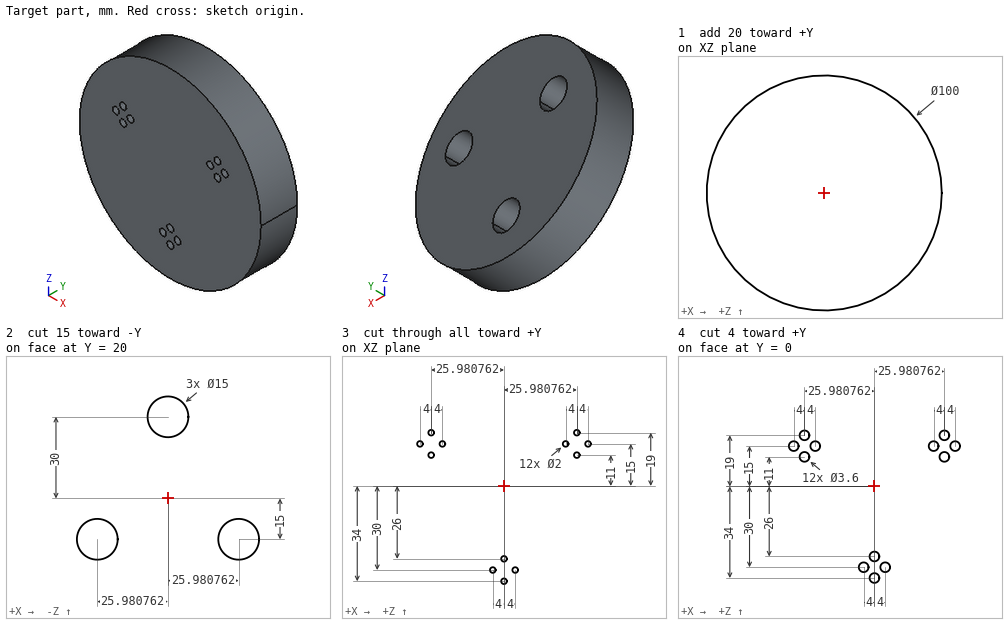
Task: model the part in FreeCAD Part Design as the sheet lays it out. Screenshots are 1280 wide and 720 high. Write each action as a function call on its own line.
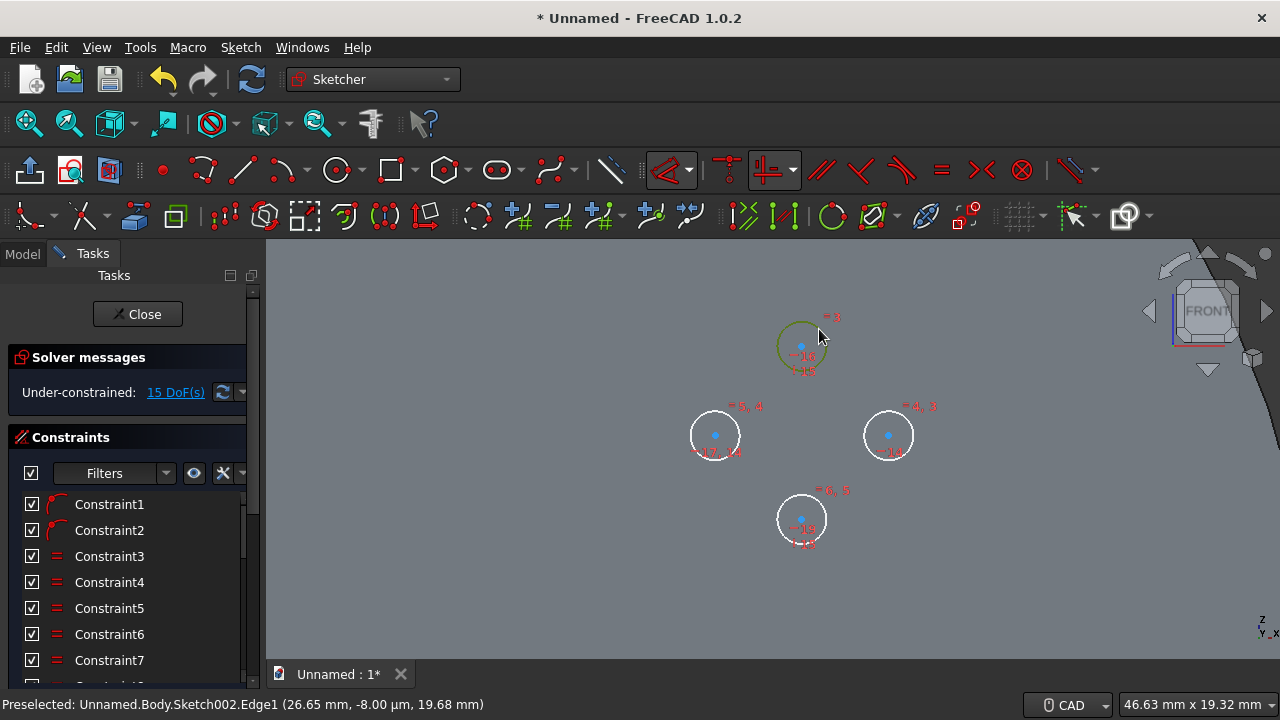
click(692, 170)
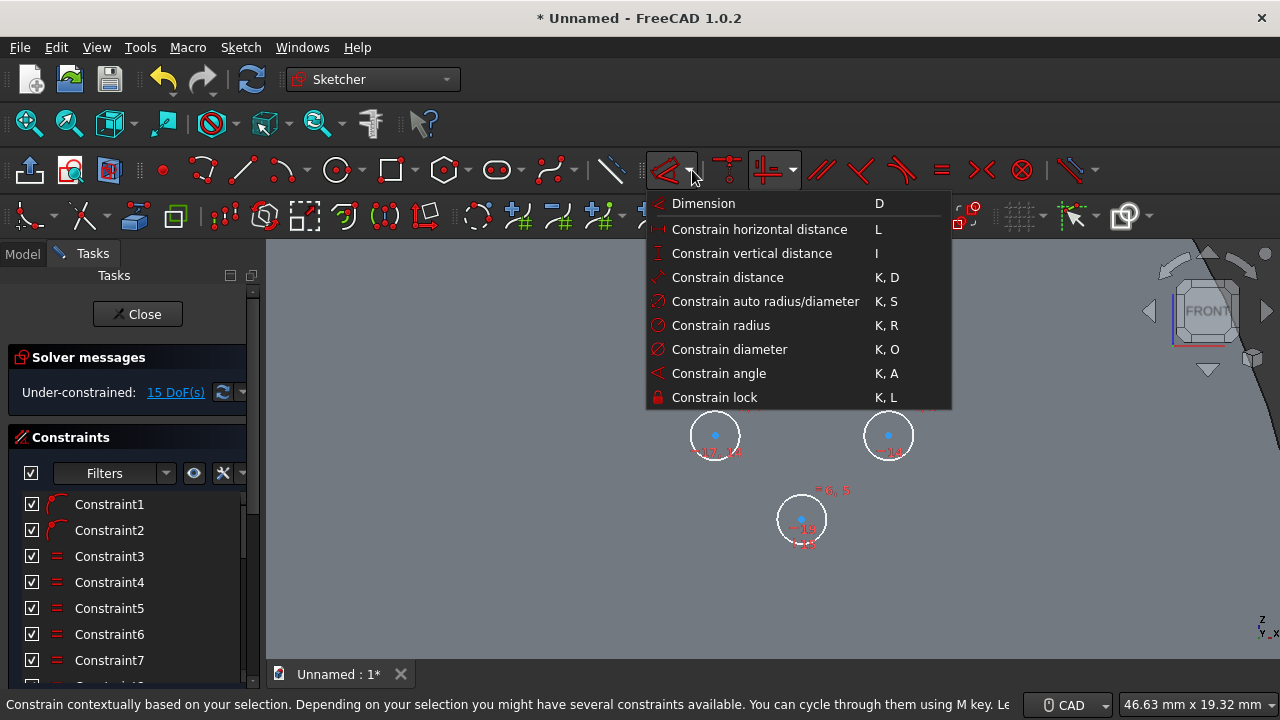
click(799, 349)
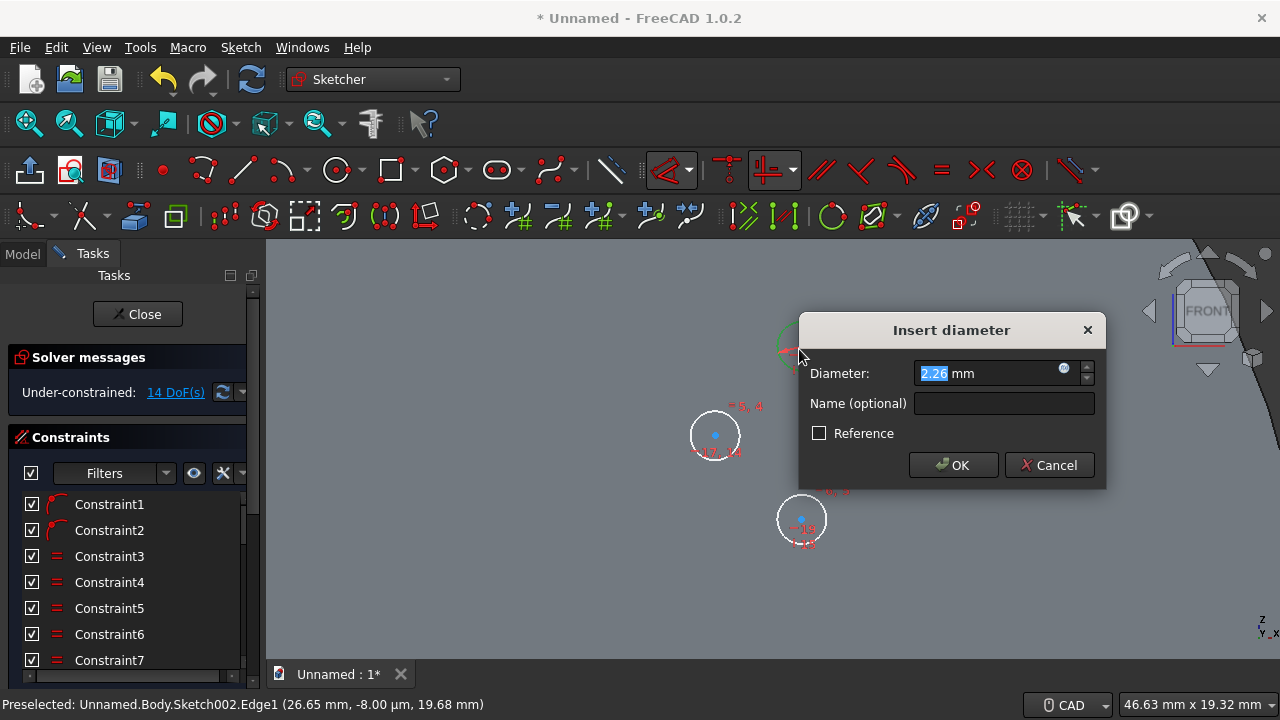
text(2)
key(Return)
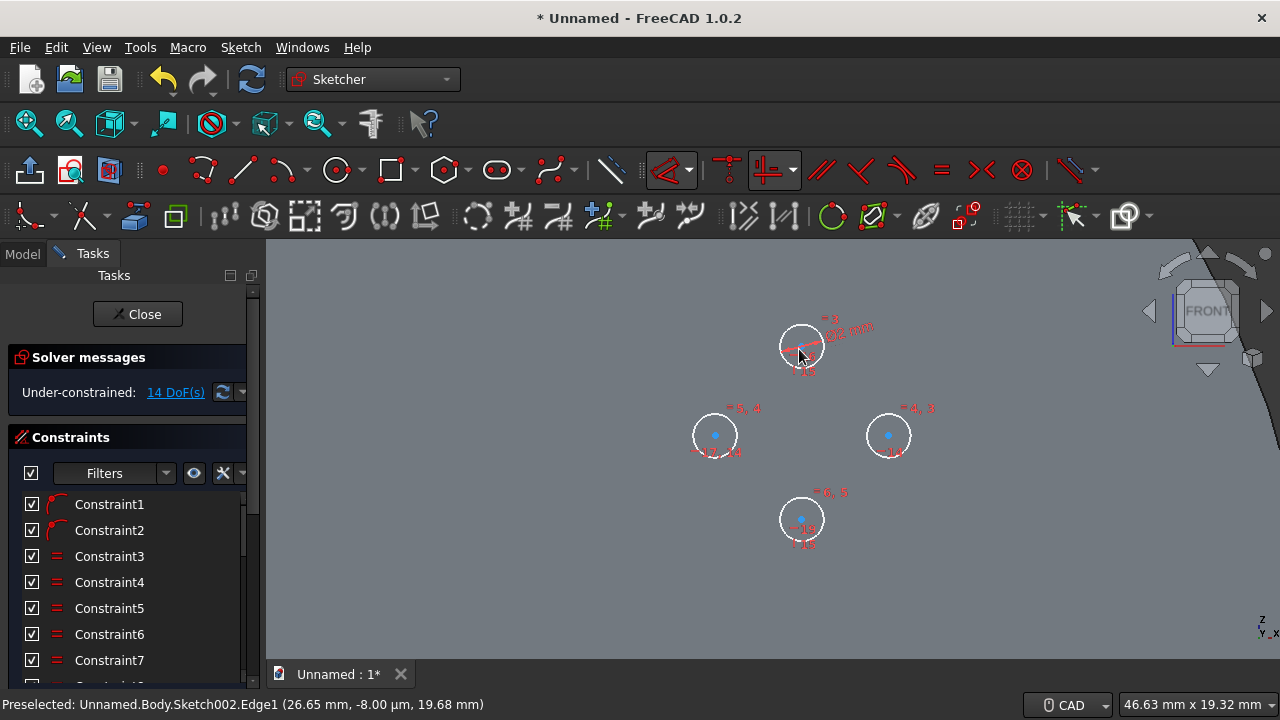
scroll(822, 330, down, 8)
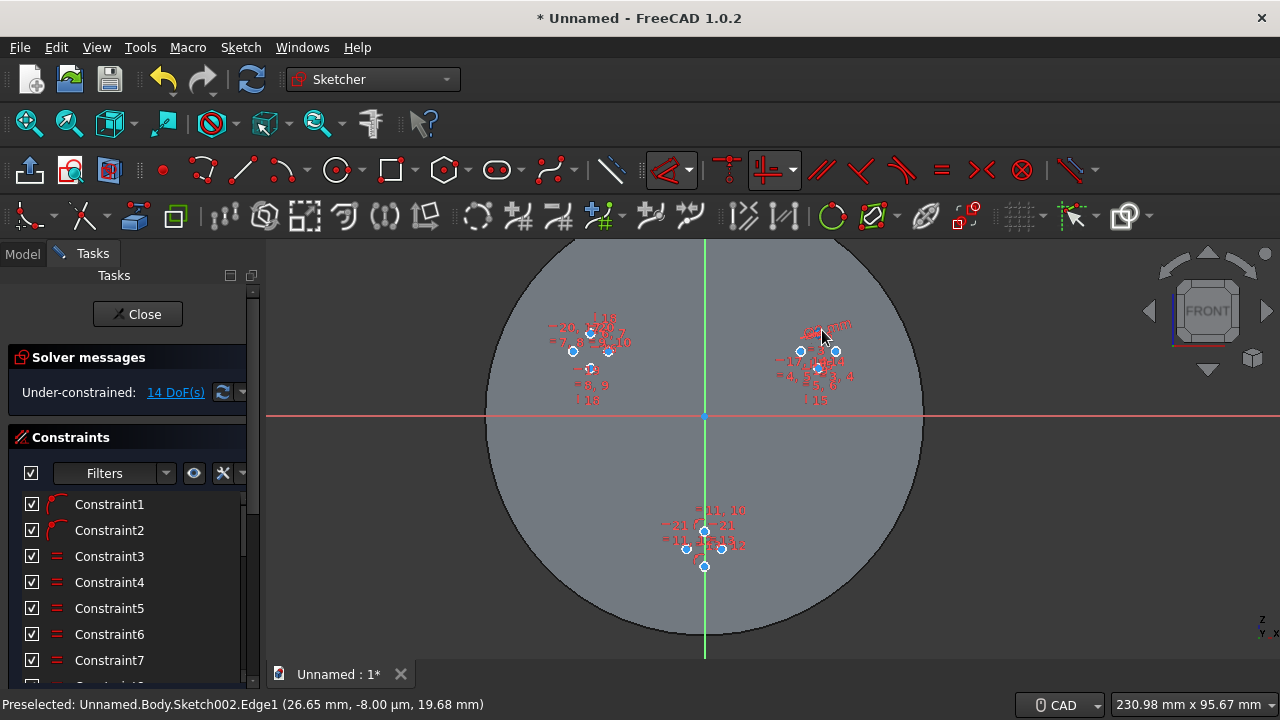
scroll(687, 549, up, 5)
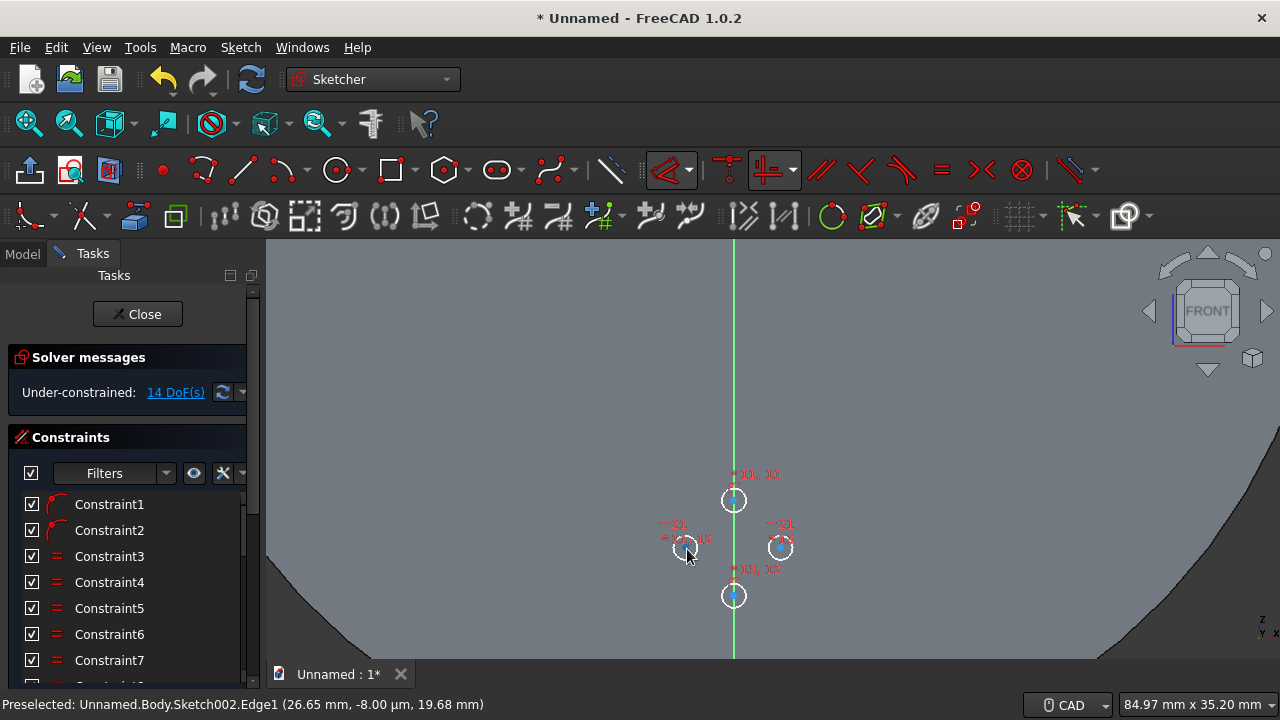
click(685, 548)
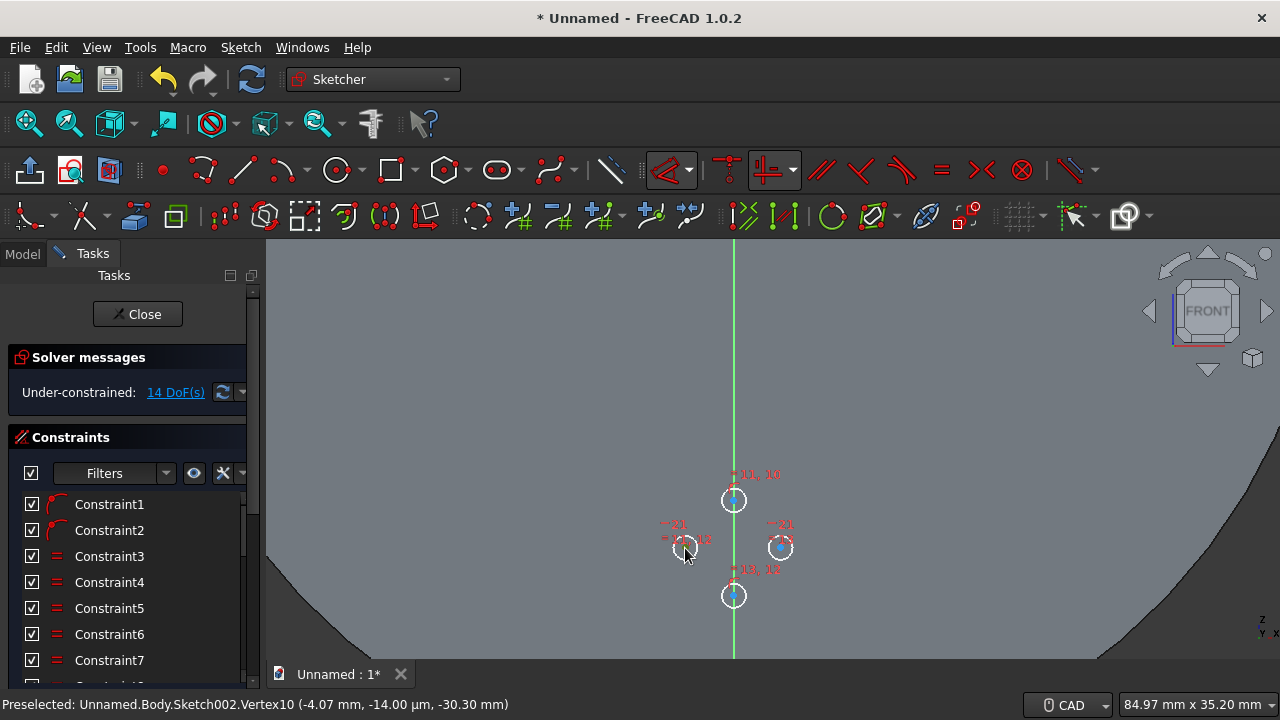
click(692, 170)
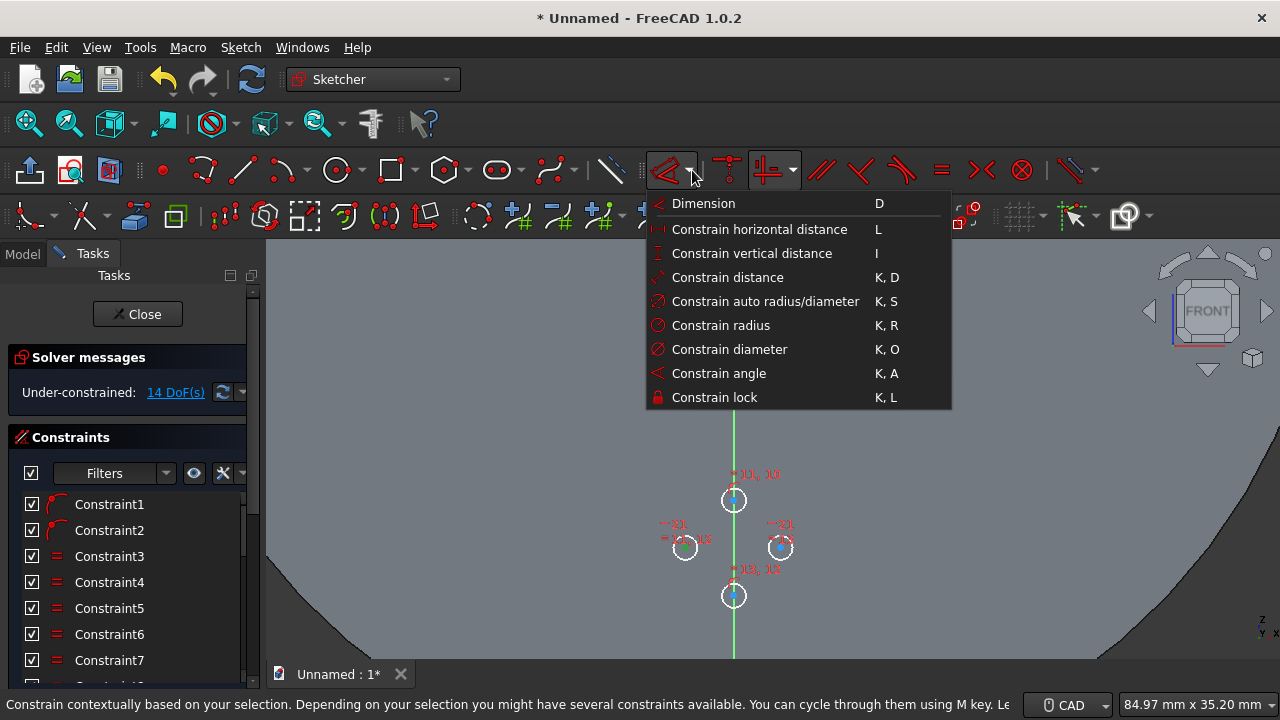
click(799, 229)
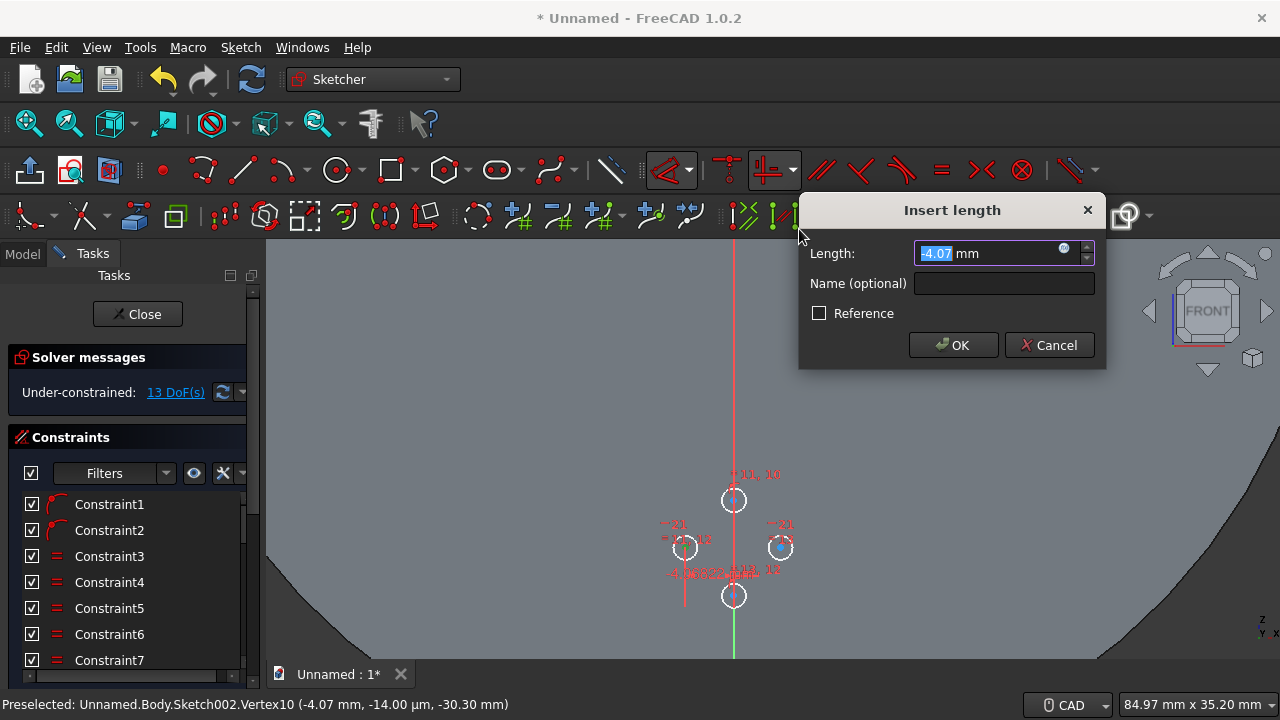
text(-4)
key(Return)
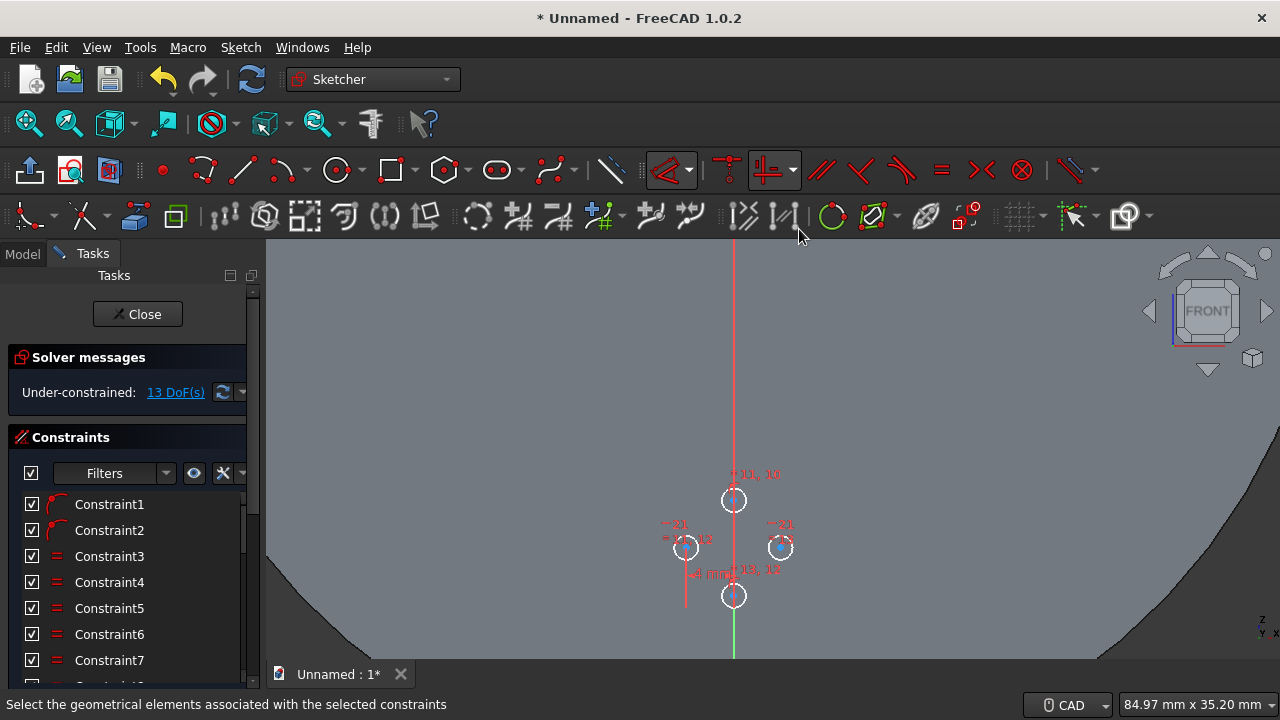
click(781, 548)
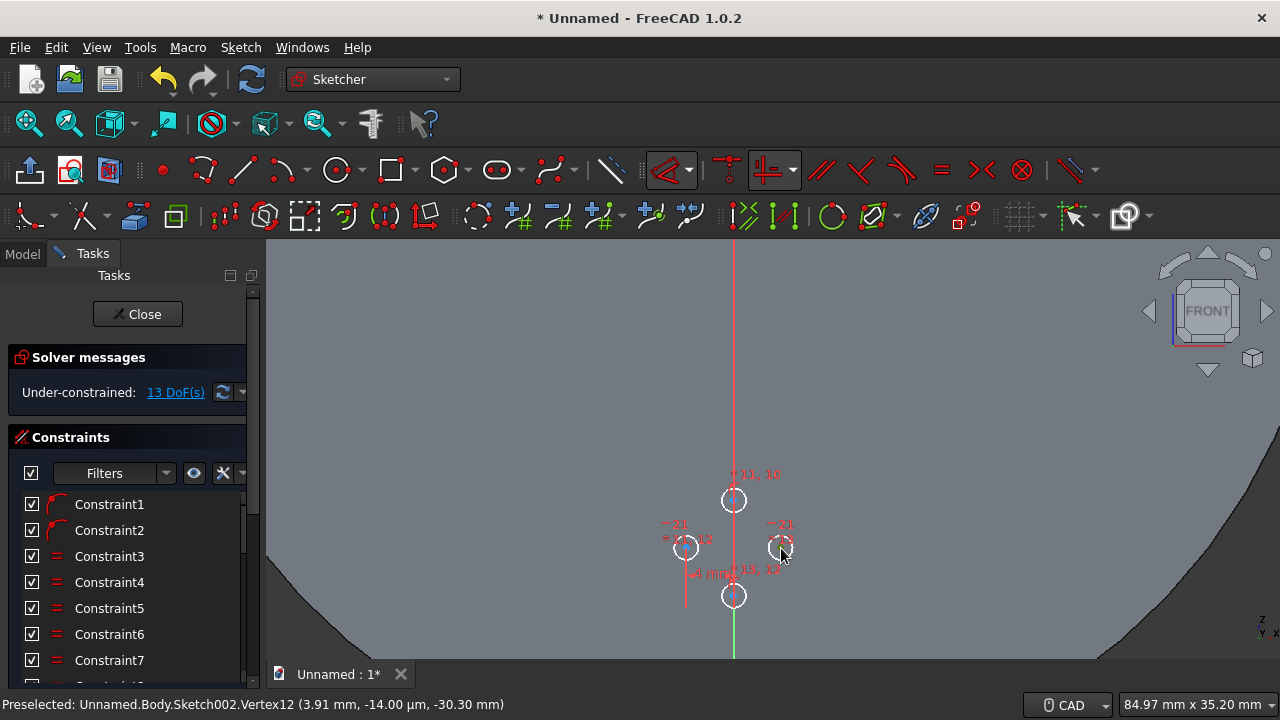
key(l)